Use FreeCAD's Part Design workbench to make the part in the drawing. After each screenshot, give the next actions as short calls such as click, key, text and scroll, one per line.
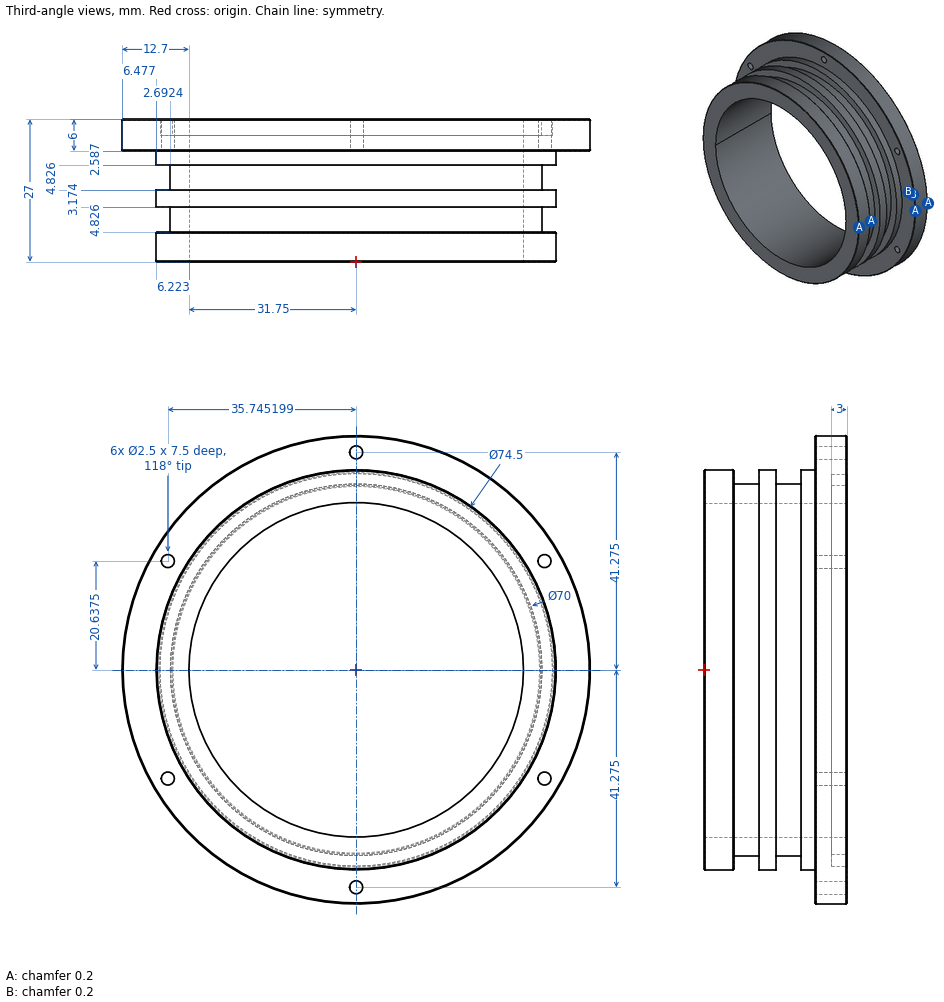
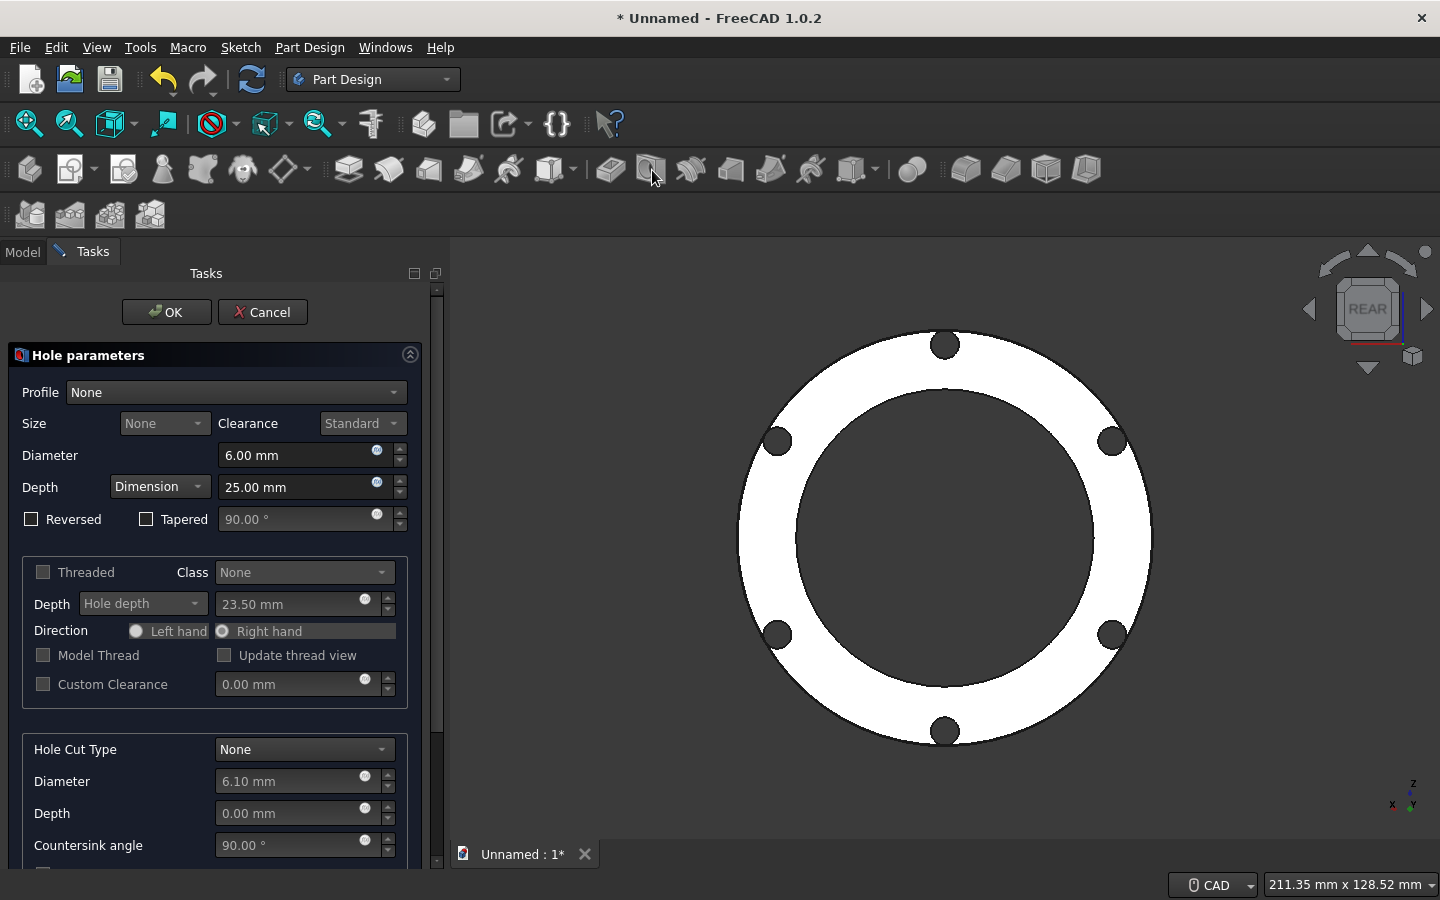
triple_click(305, 455)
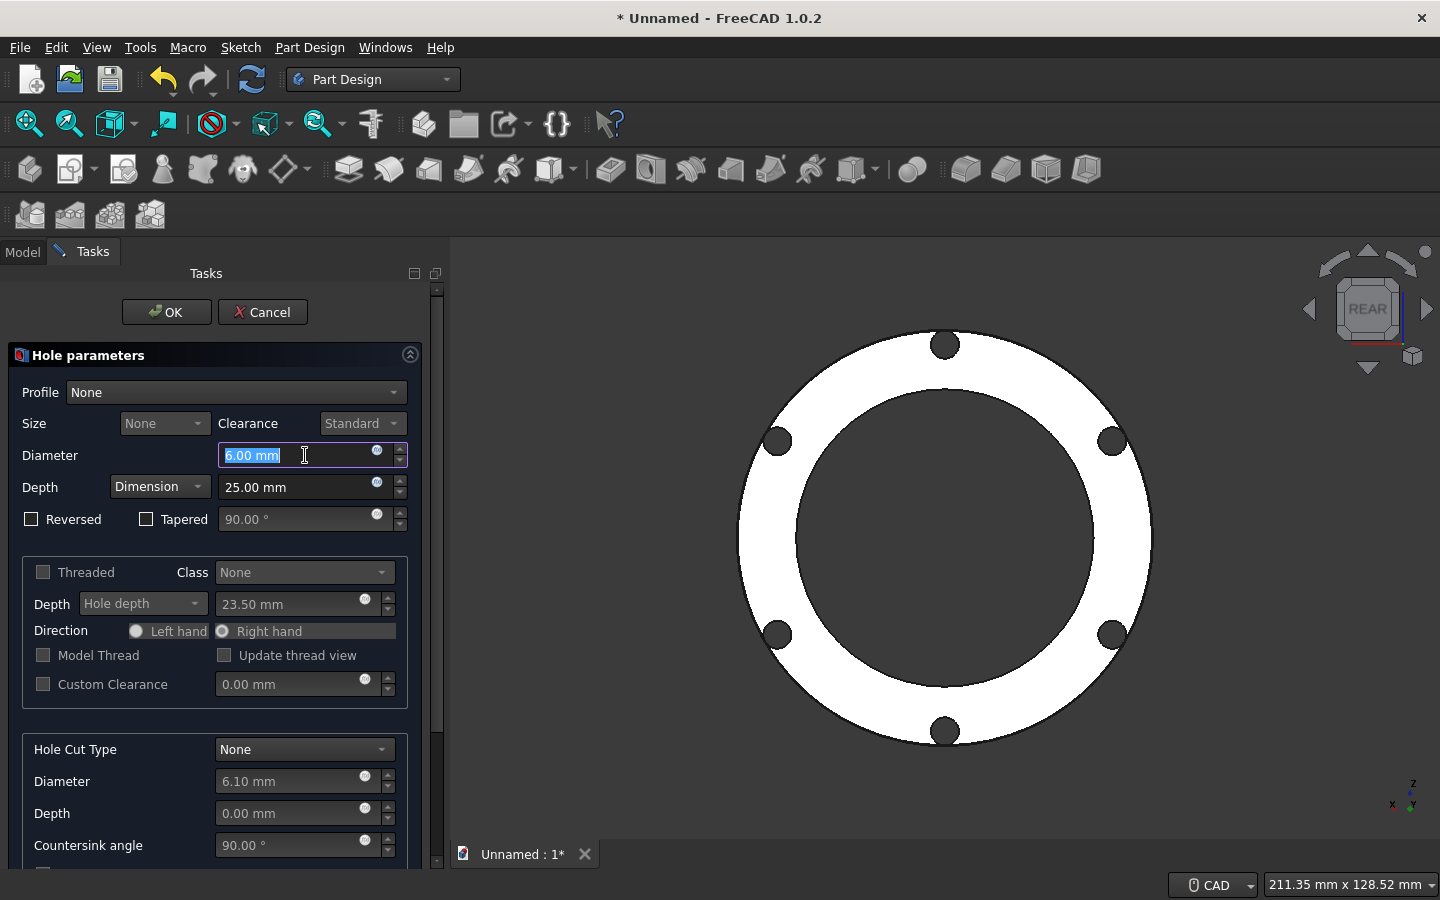
text(2.5)
key(Tab)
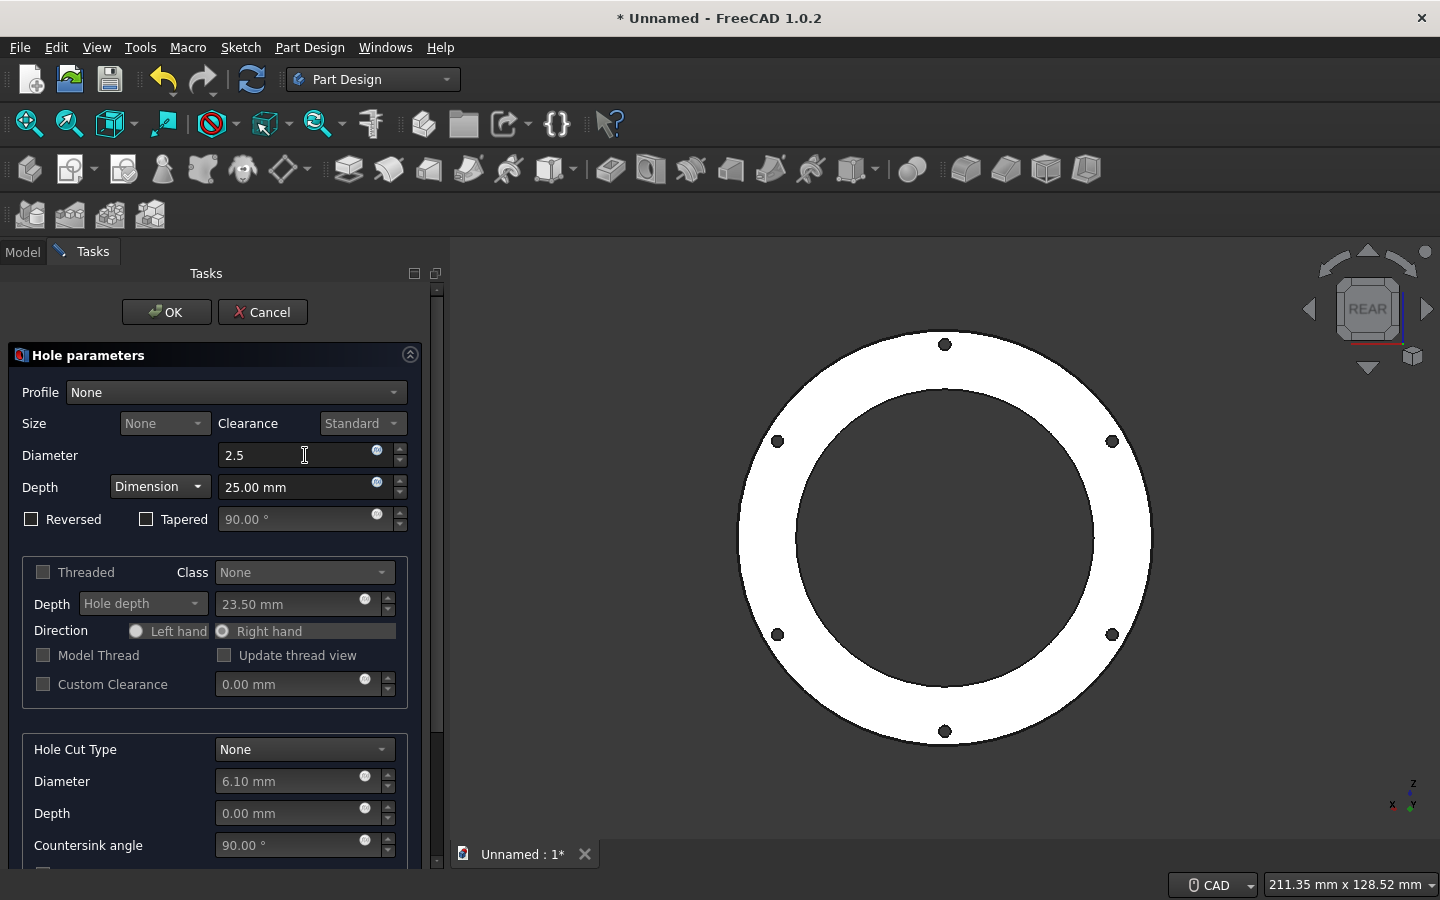
triple_click(305, 487)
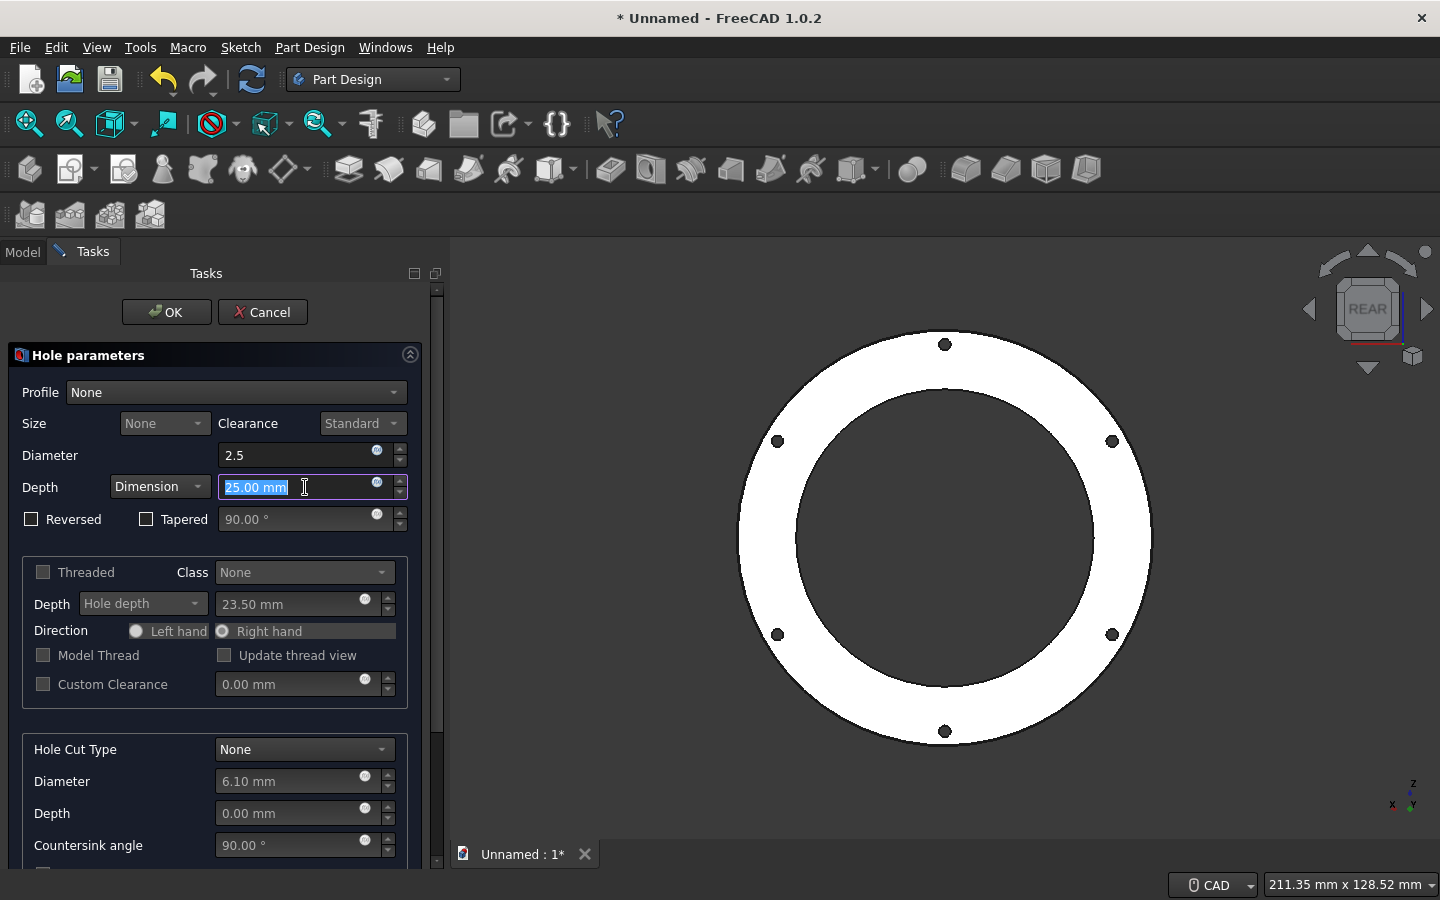
text(7.5)
key(Tab)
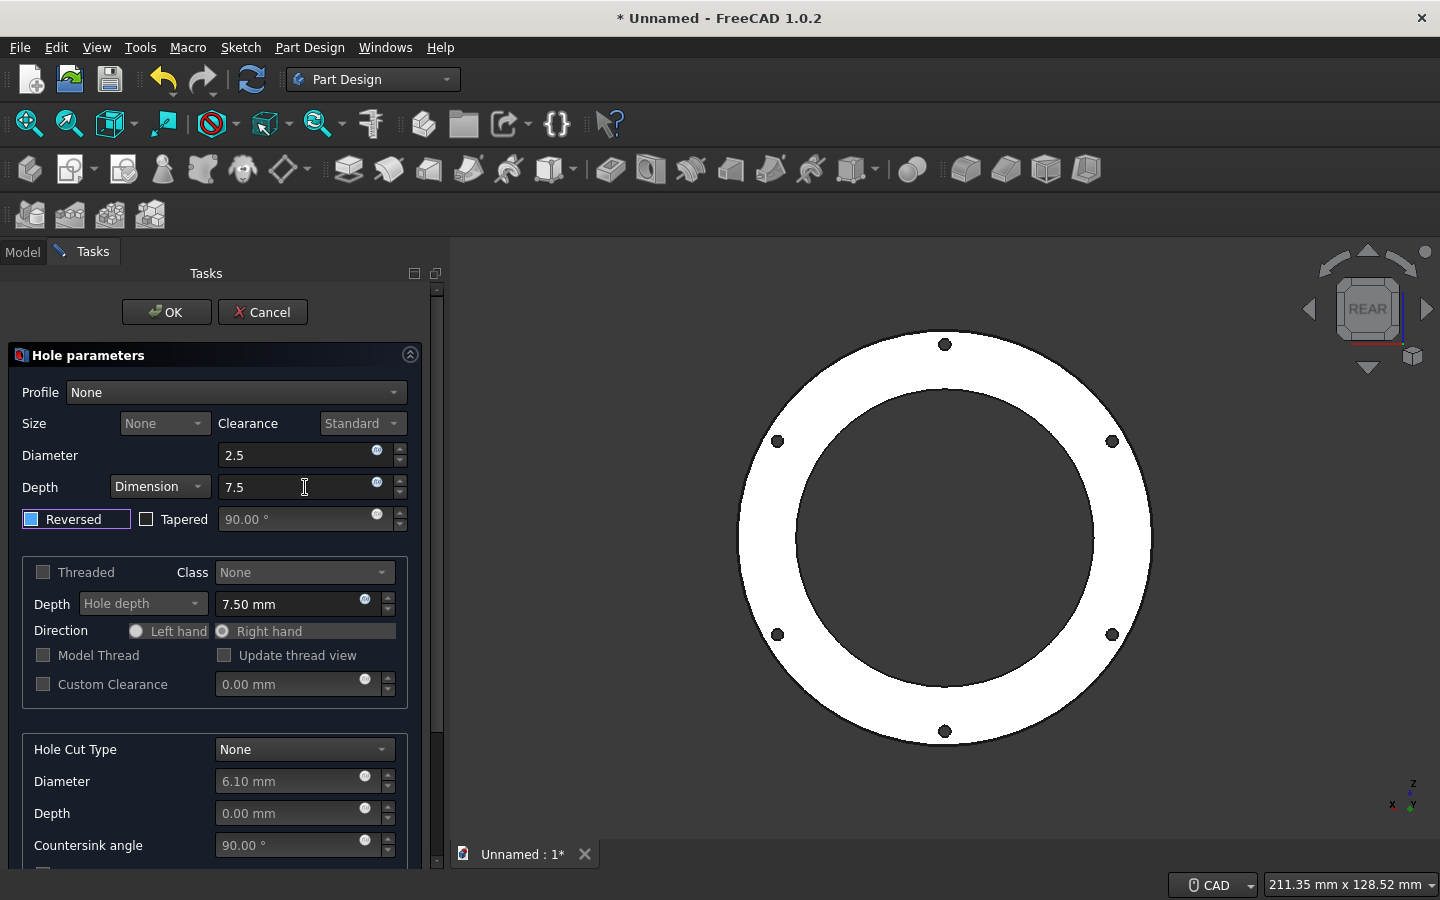
click(167, 312)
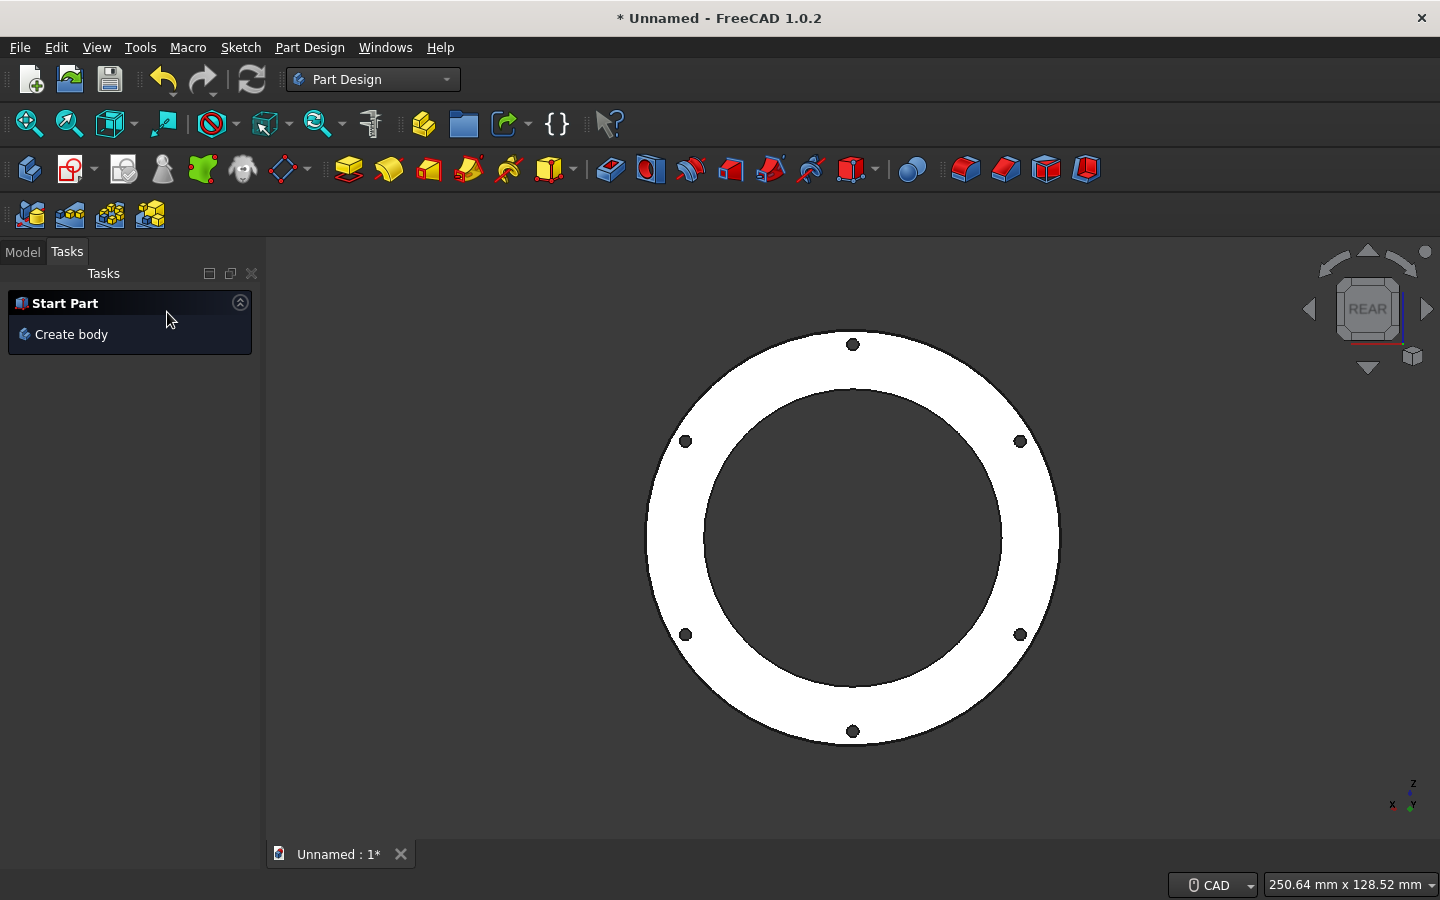
click(675, 537)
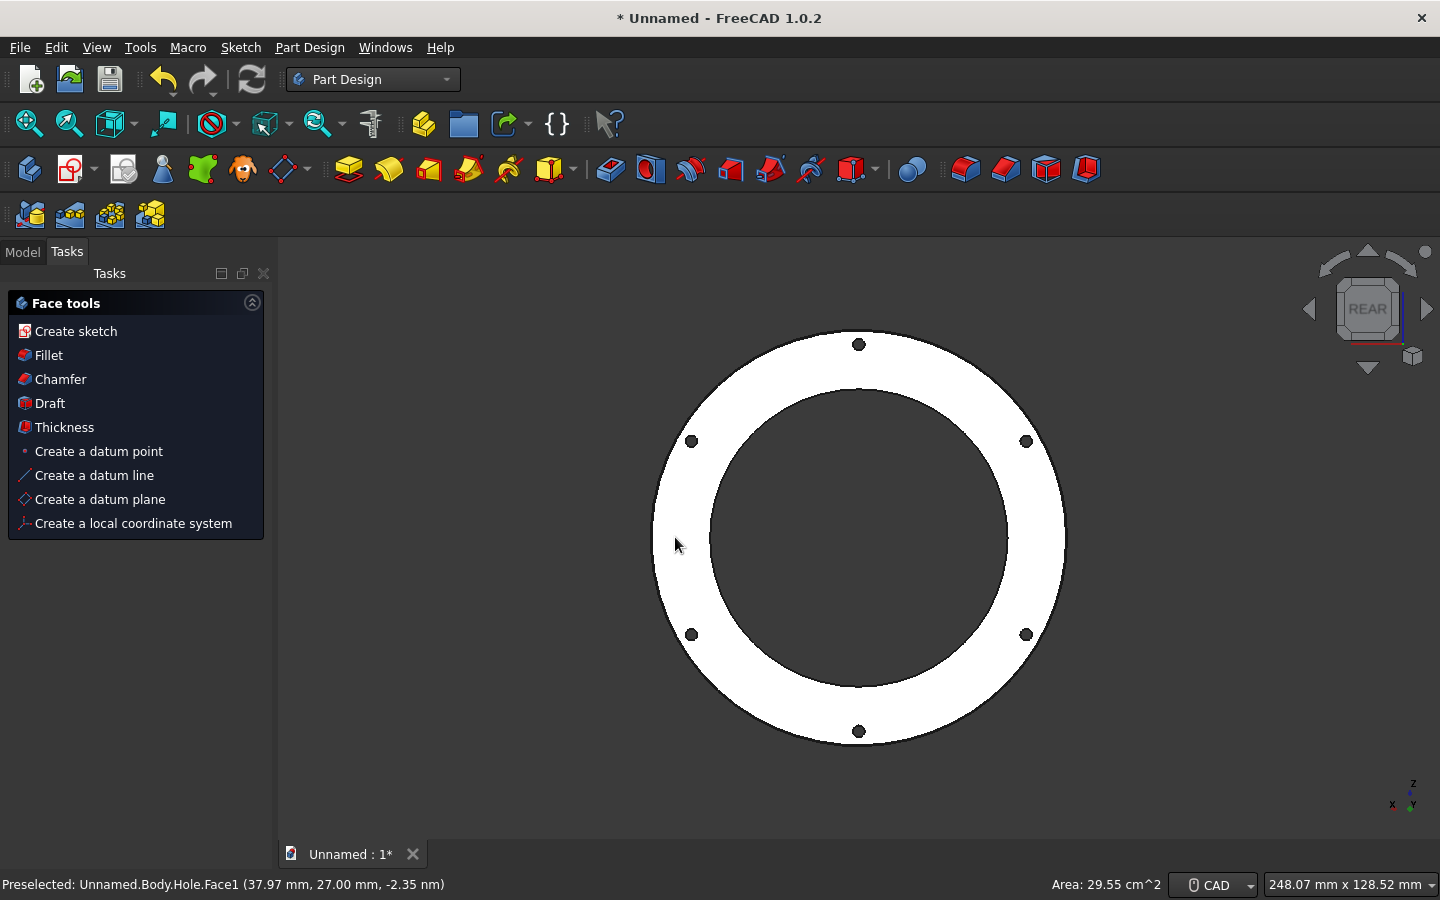
click(70, 170)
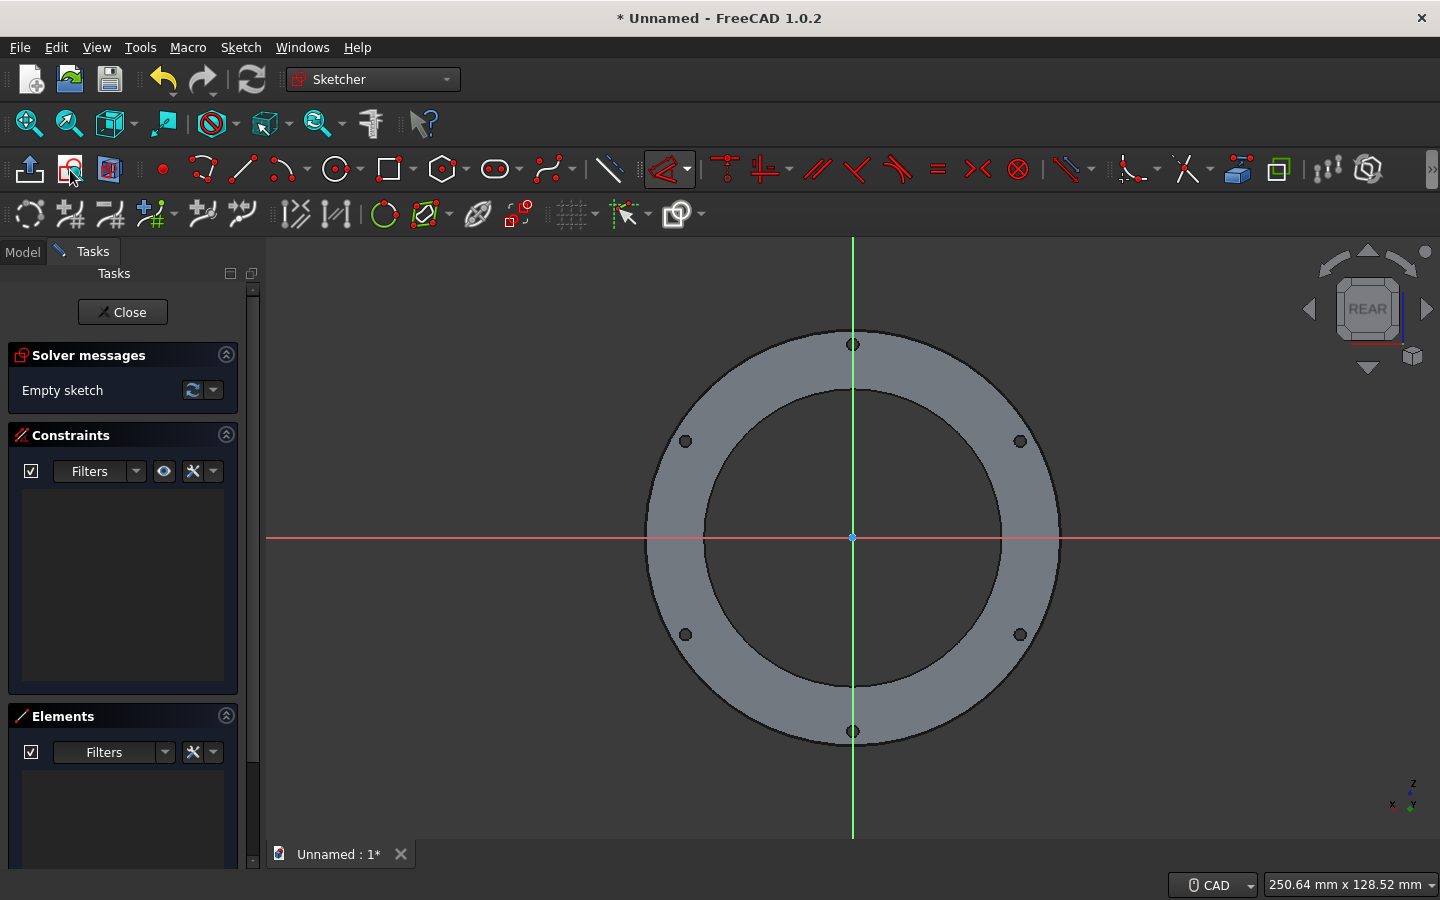
key(g)
key(c)